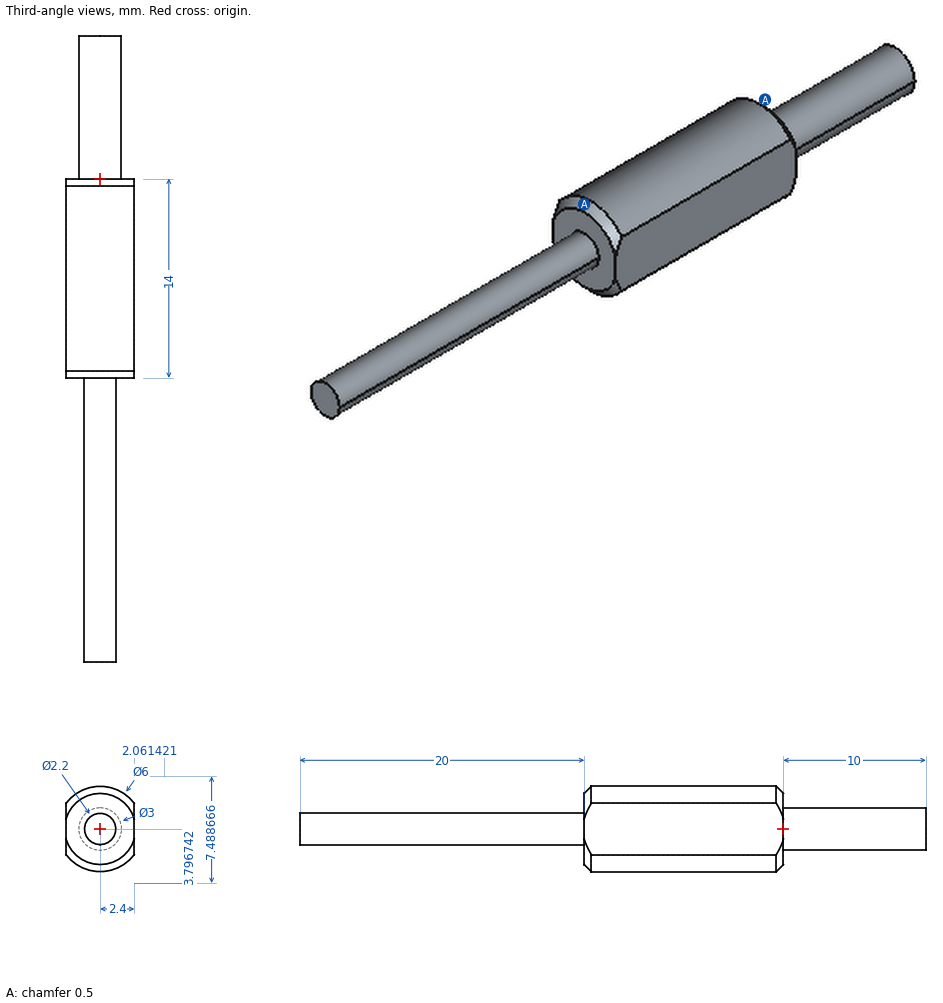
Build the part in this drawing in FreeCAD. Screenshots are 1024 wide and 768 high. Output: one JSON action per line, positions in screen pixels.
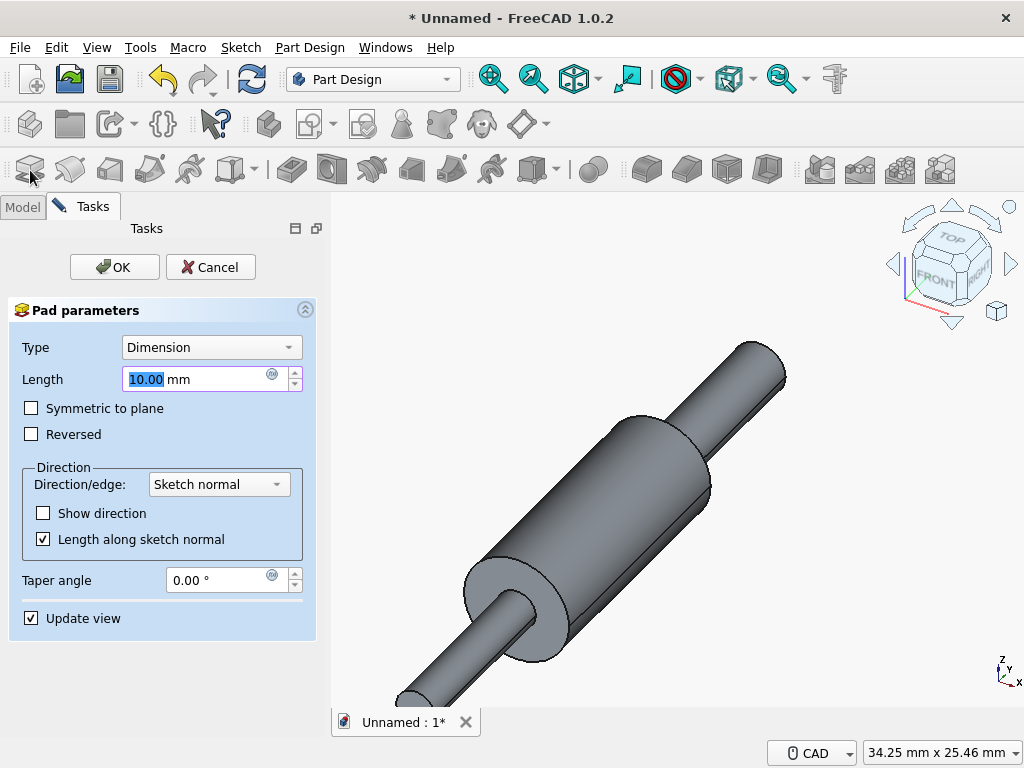
{"action": "type", "text": "20"}
{"action": "key", "text": "Tab"}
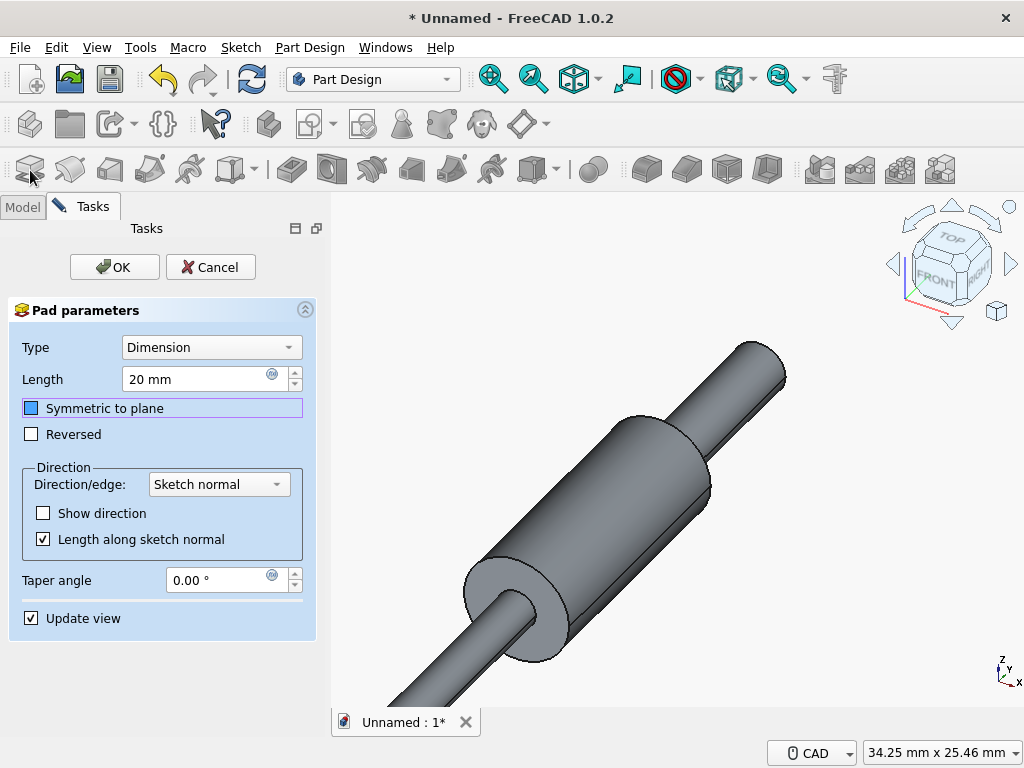
{"action": "left_click", "coordinate": [115, 267]}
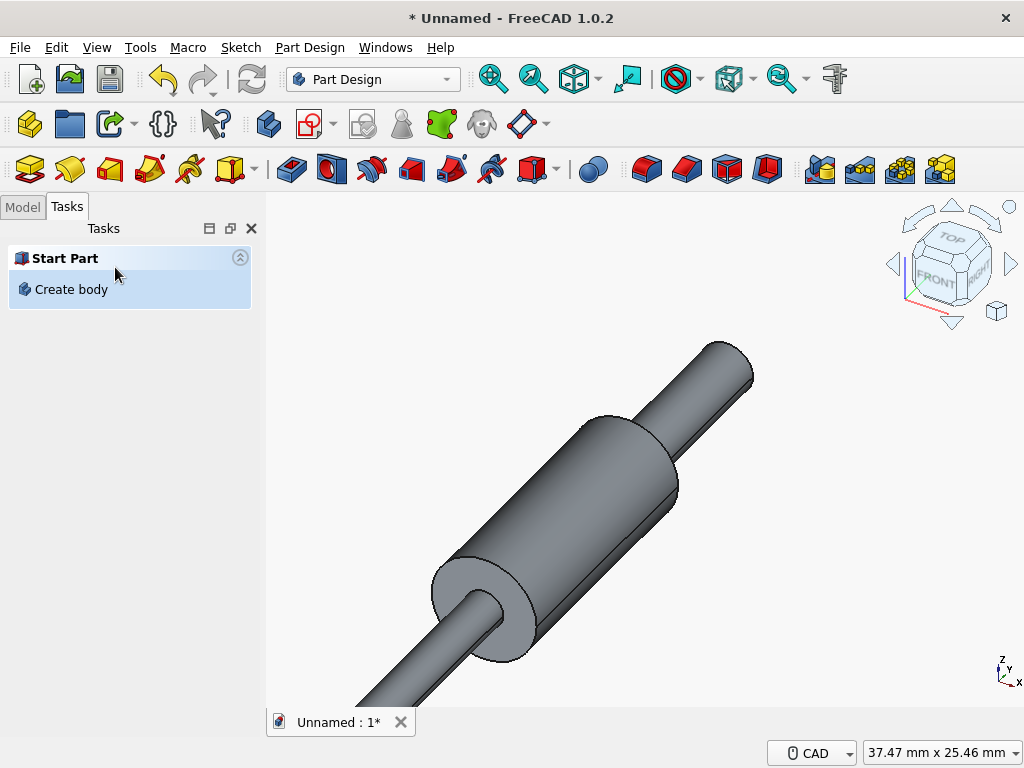
{"action": "left_click", "coordinate": [494, 80]}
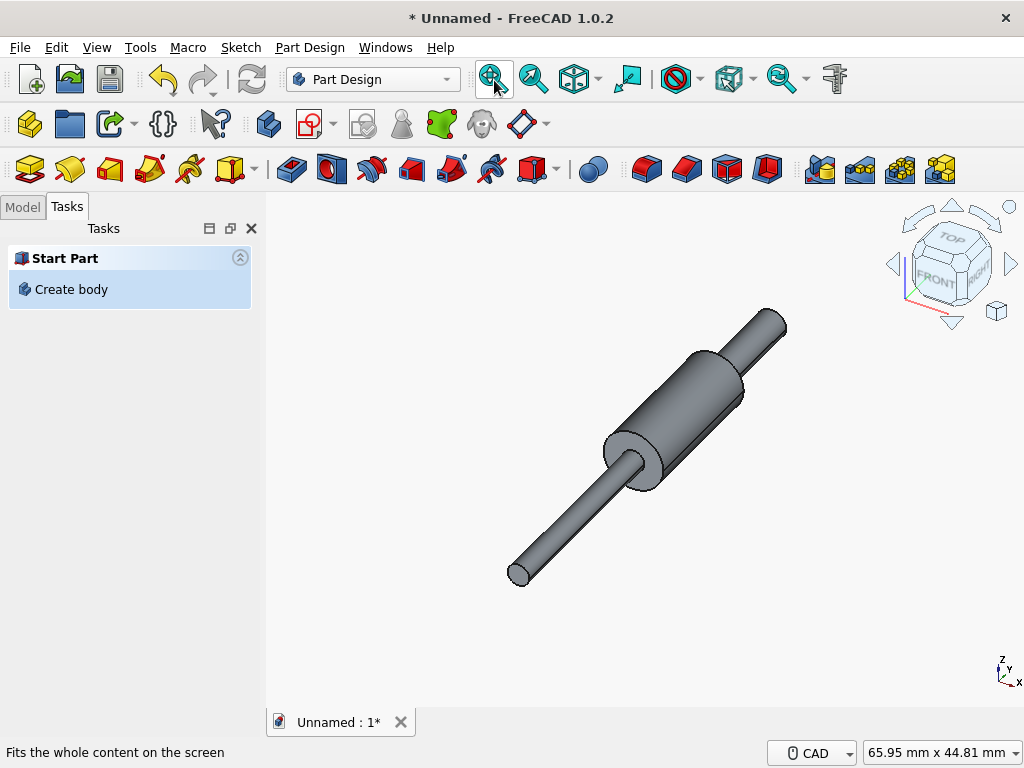
{"action": "left_click", "coordinate": [609, 435]}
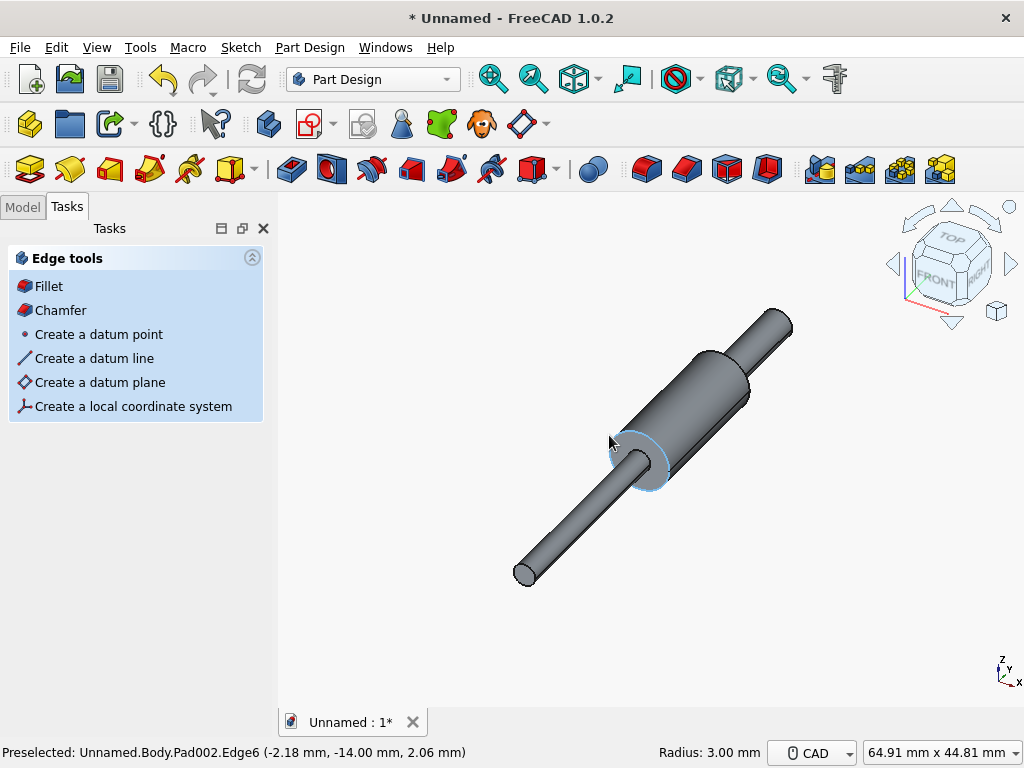
{"action": "key", "text": "0"}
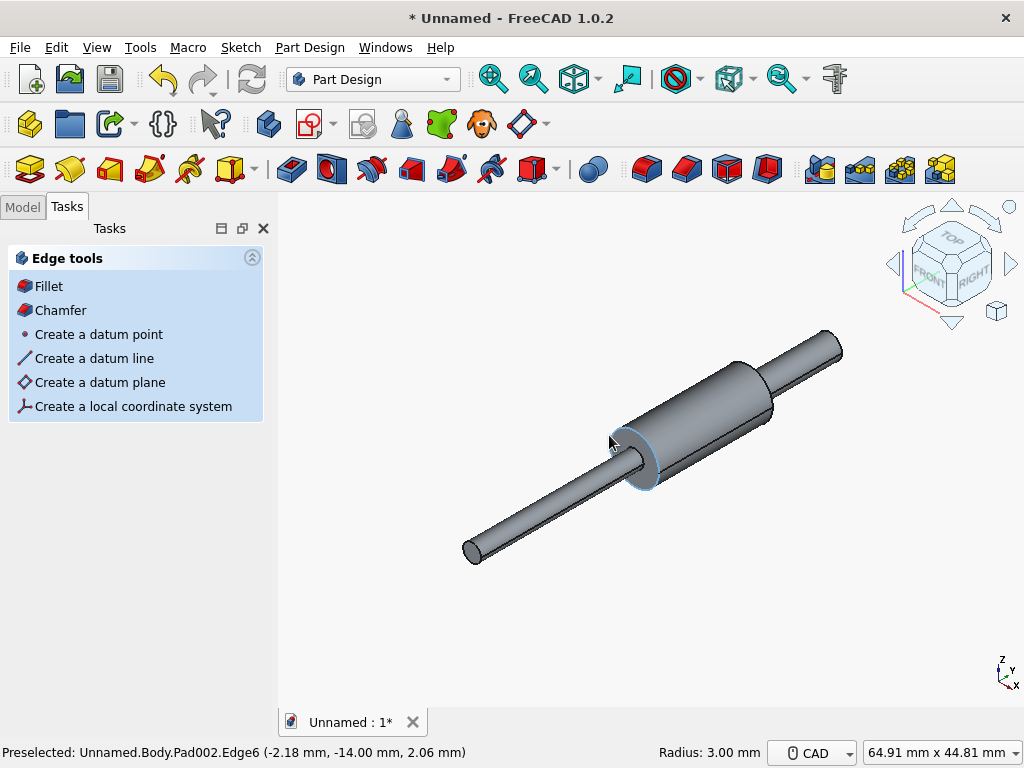
{"action": "key", "text": "2"}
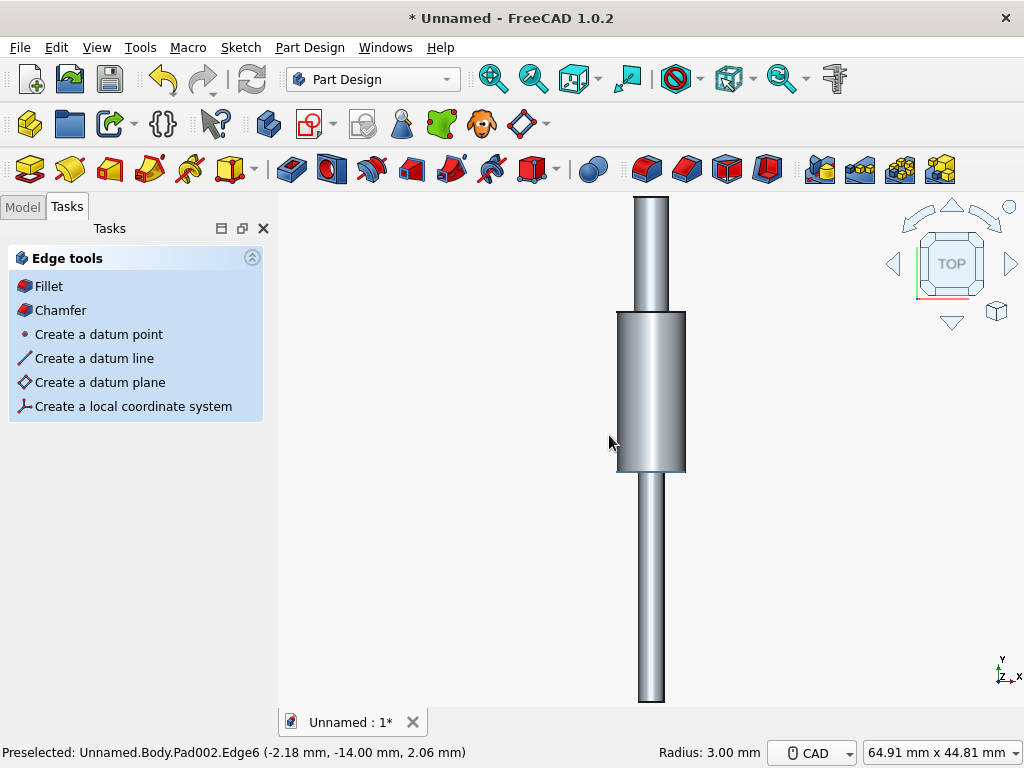
{"action": "left_click", "coordinate": [623, 311], "text": "ctrl"}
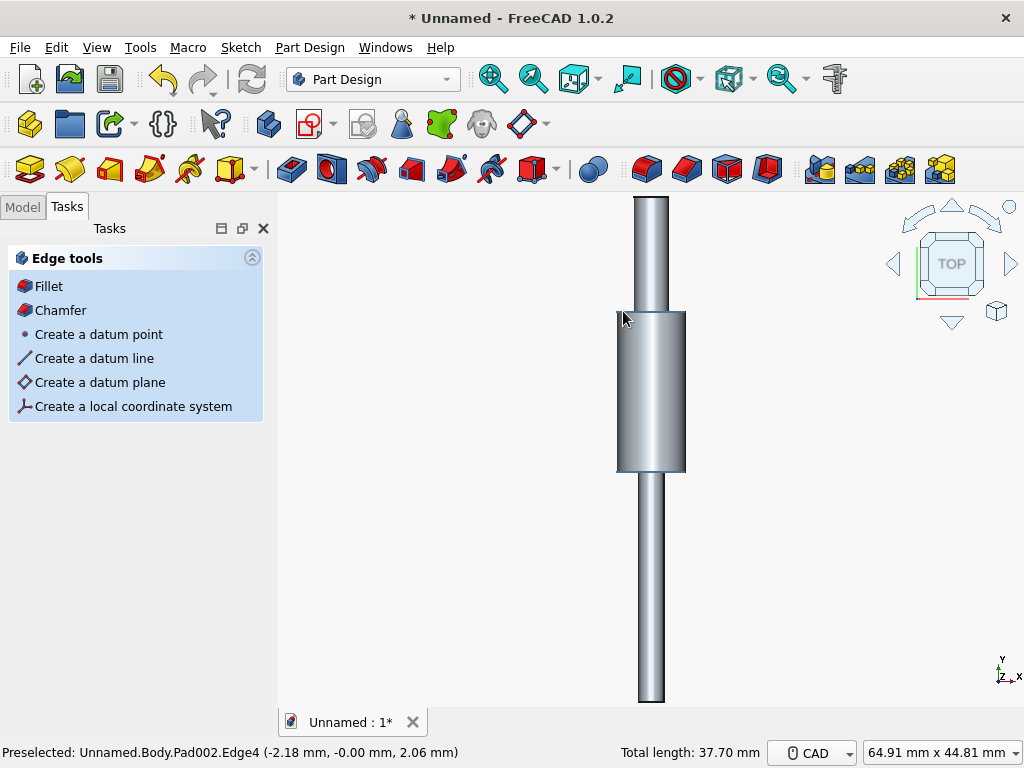
{"action": "left_click", "coordinate": [688, 170]}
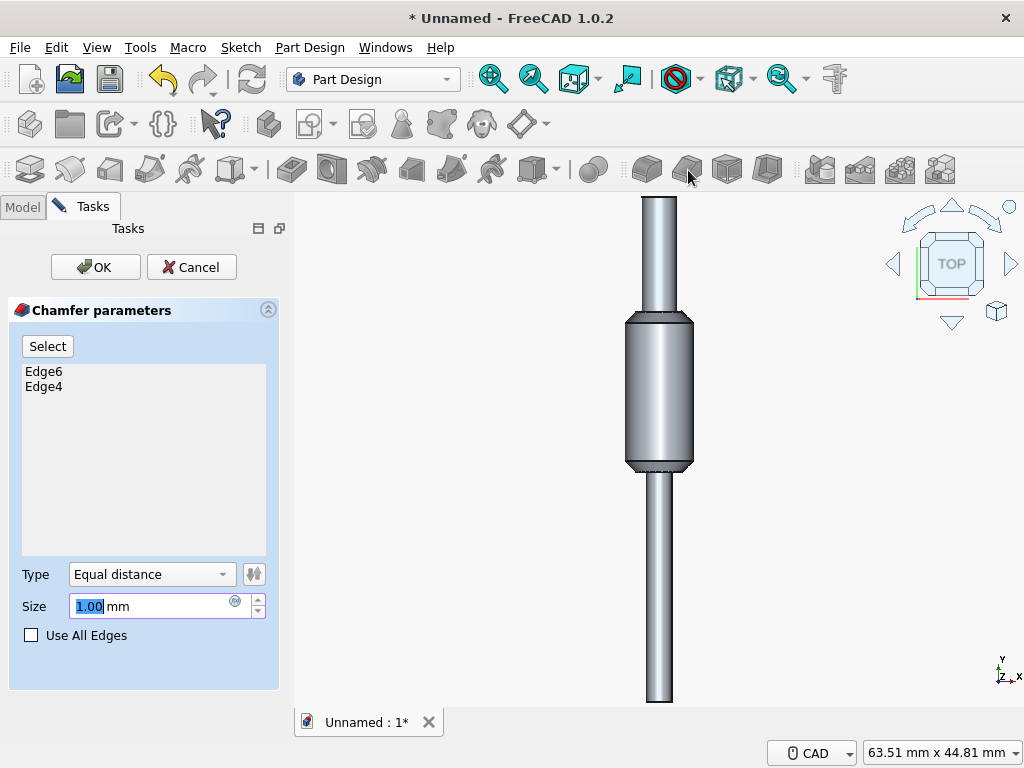
{"action": "type", "text": "0.5"}
{"action": "key", "text": "Tab"}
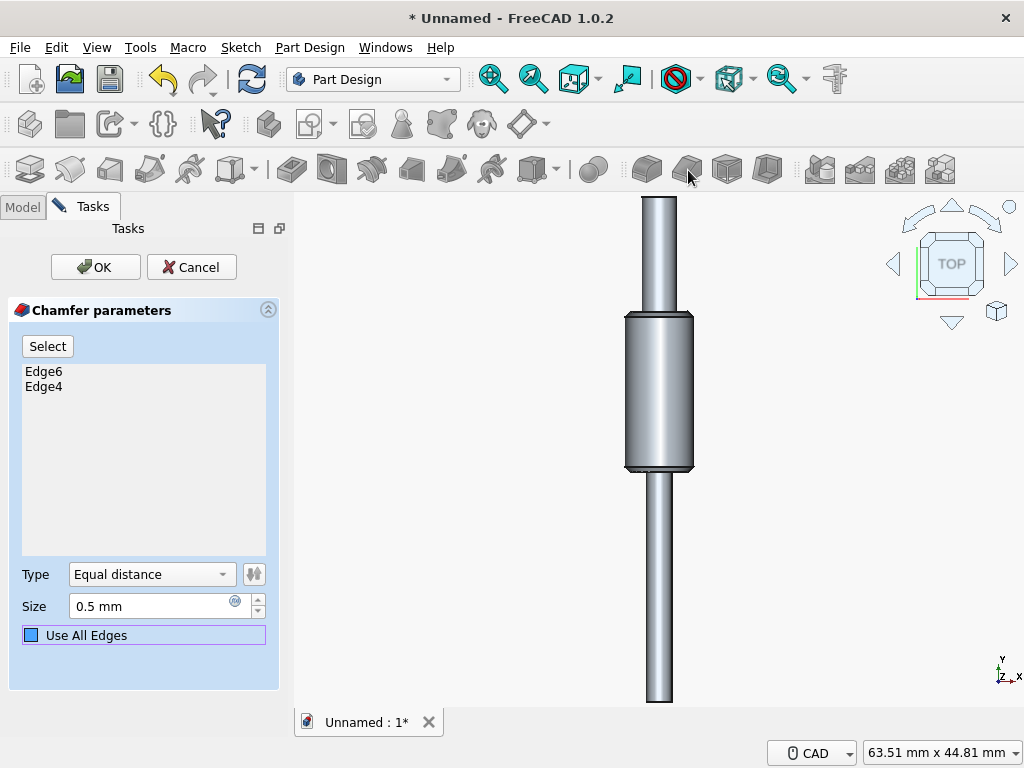
{"action": "left_click", "coordinate": [96, 267]}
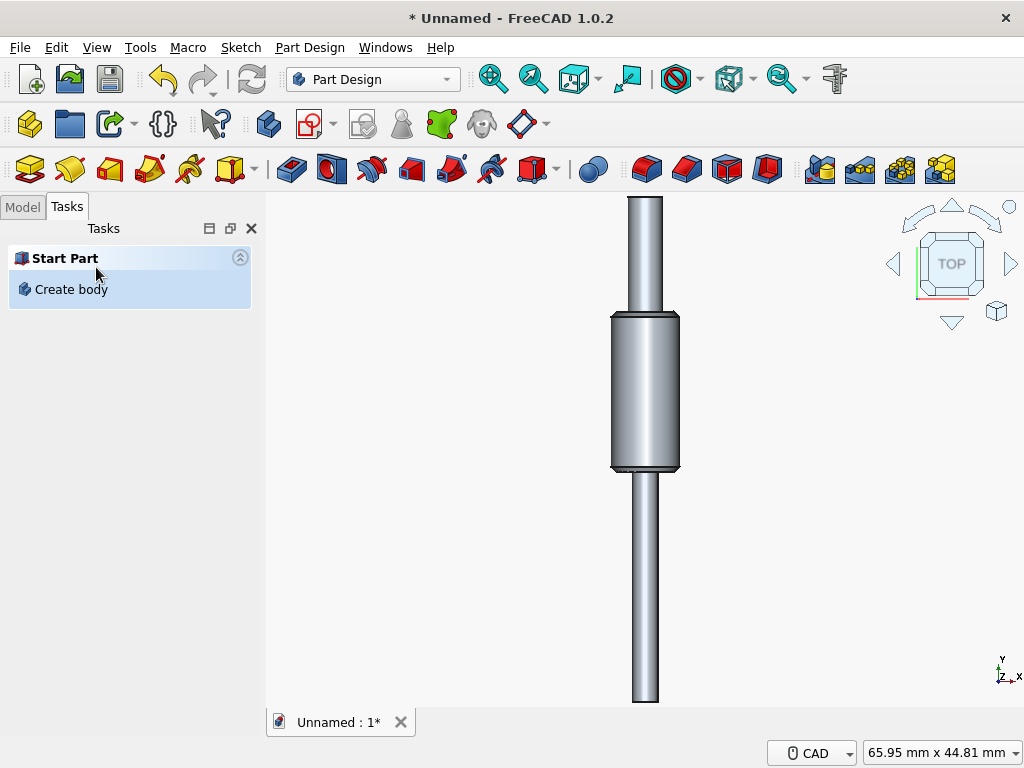
{"action": "key", "text": "4"}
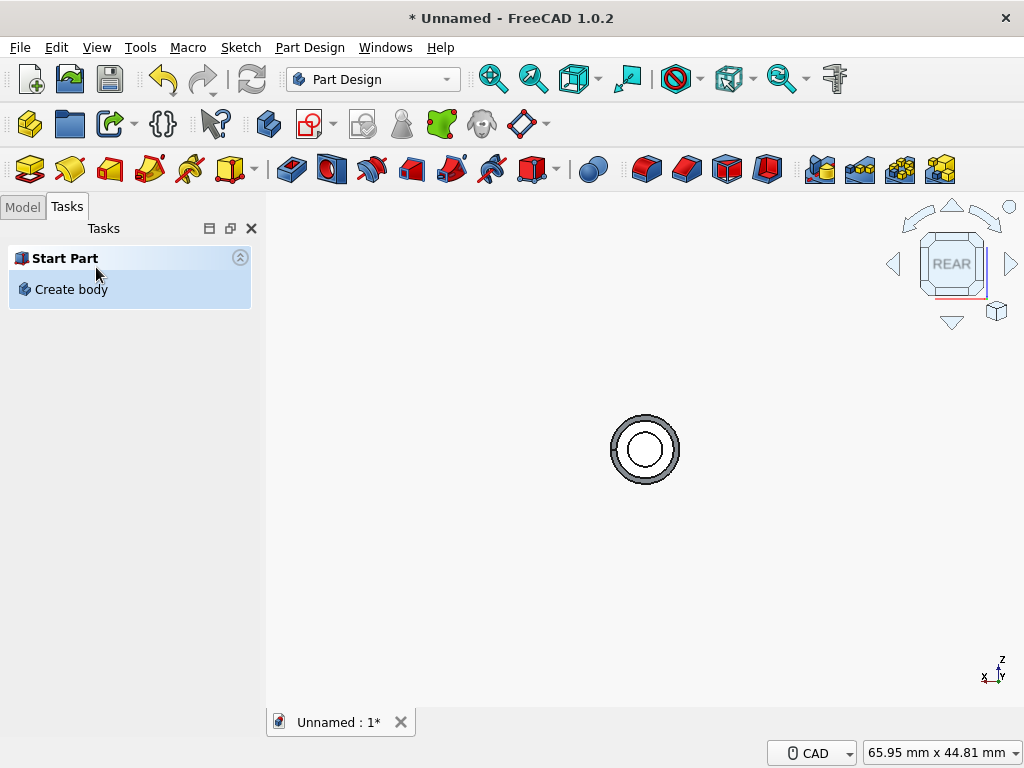
{"action": "key", "text": "v f"}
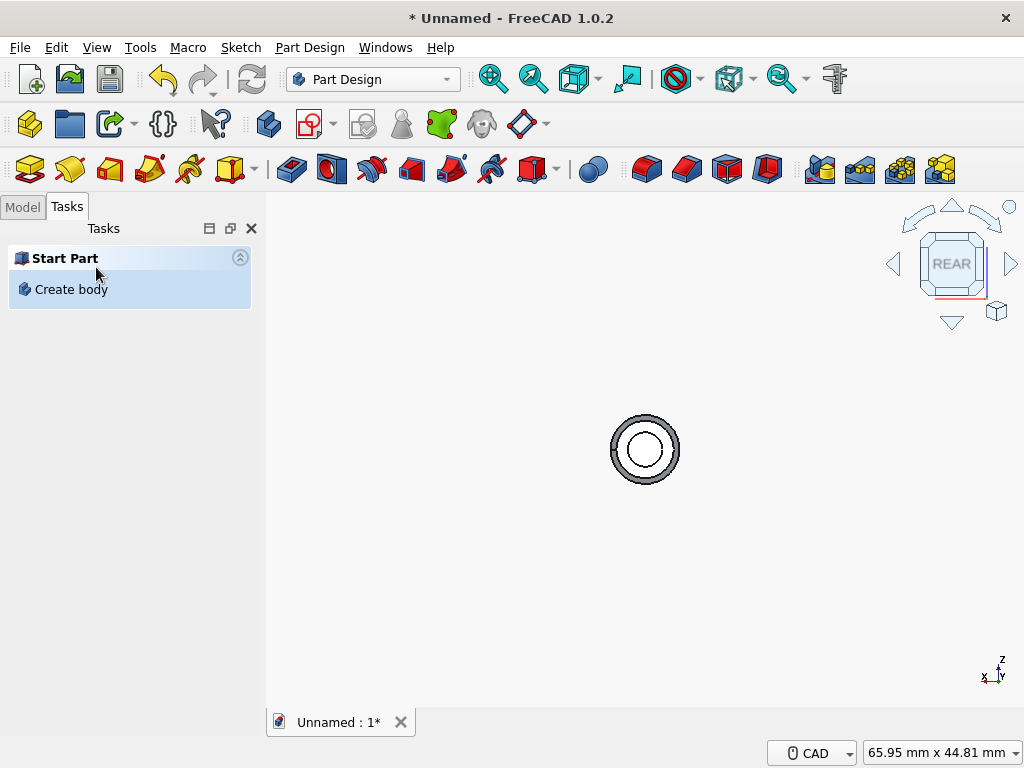
{"action": "left_click", "coordinate": [645, 448]}